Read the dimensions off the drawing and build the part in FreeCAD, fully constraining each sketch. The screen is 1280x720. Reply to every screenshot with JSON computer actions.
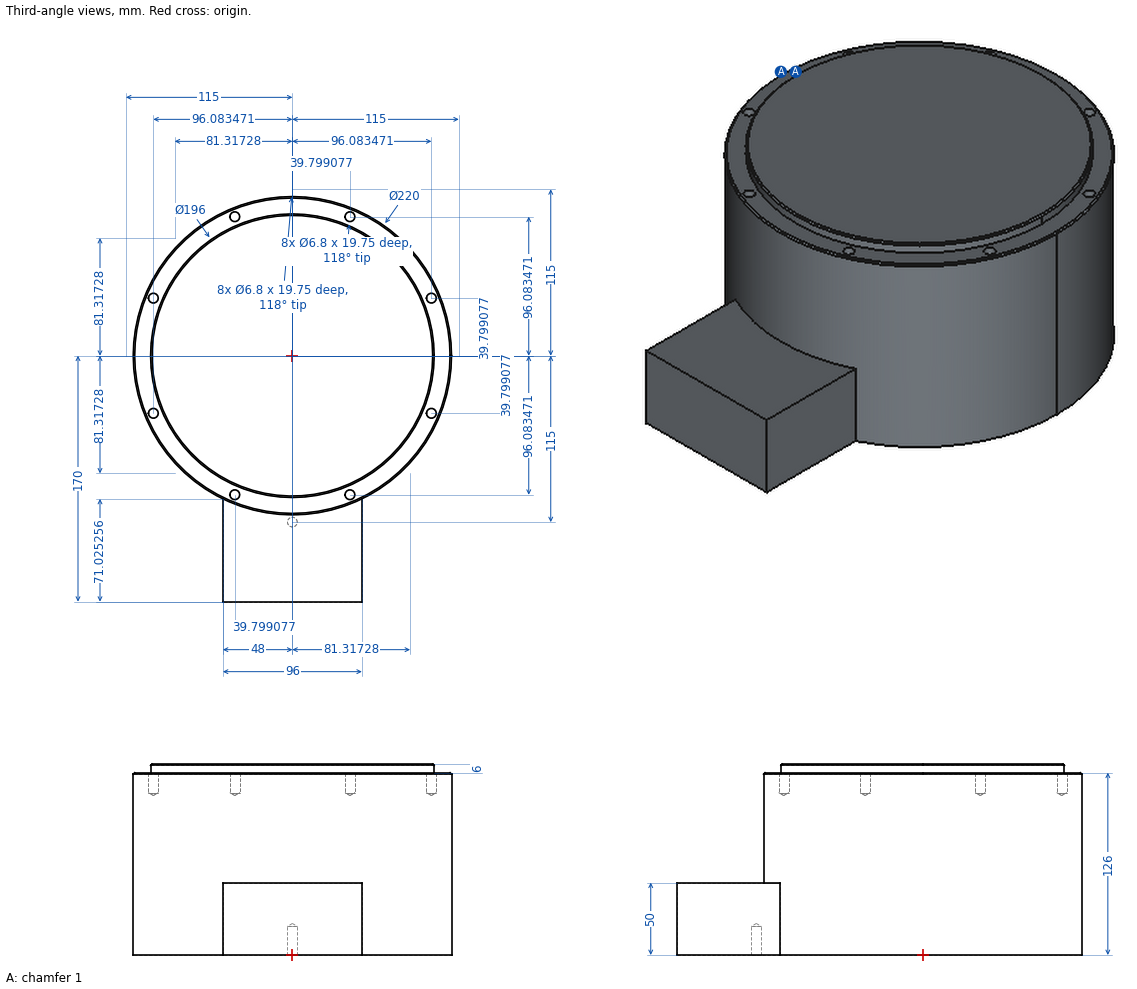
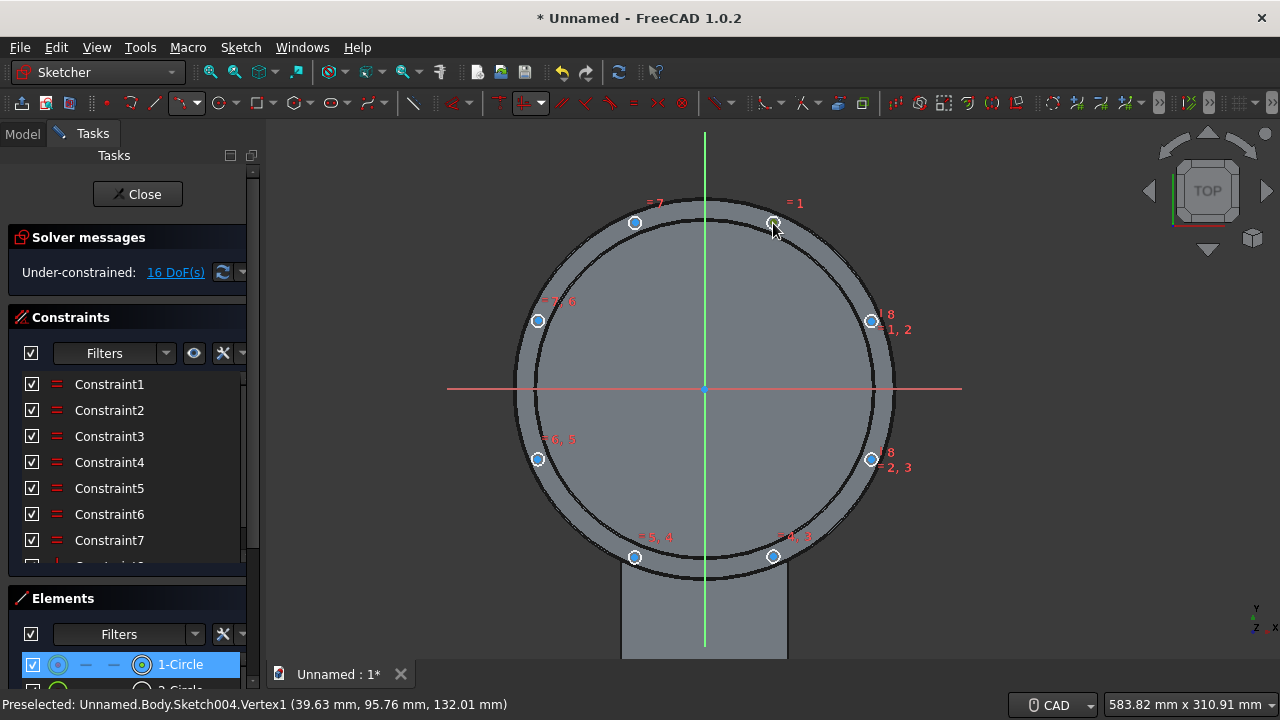
{"action": "left_click", "coordinate": [773, 557]}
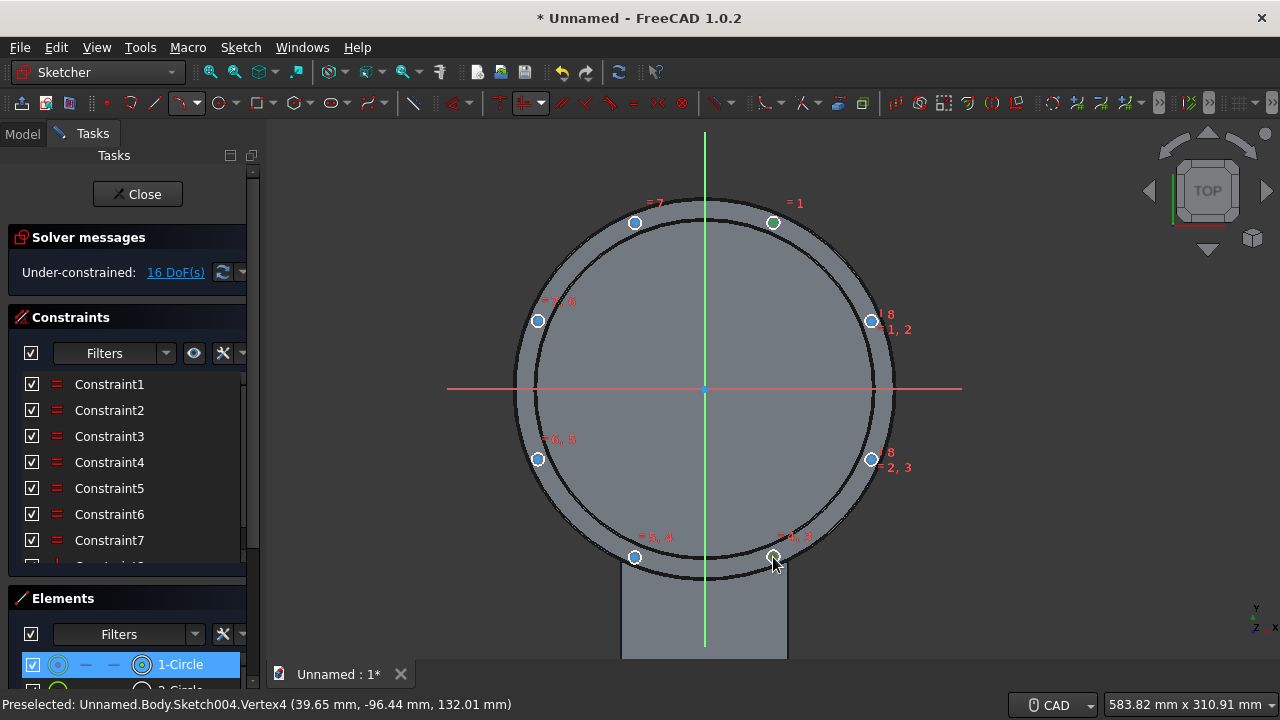
{"action": "left_click", "coordinate": [544, 104]}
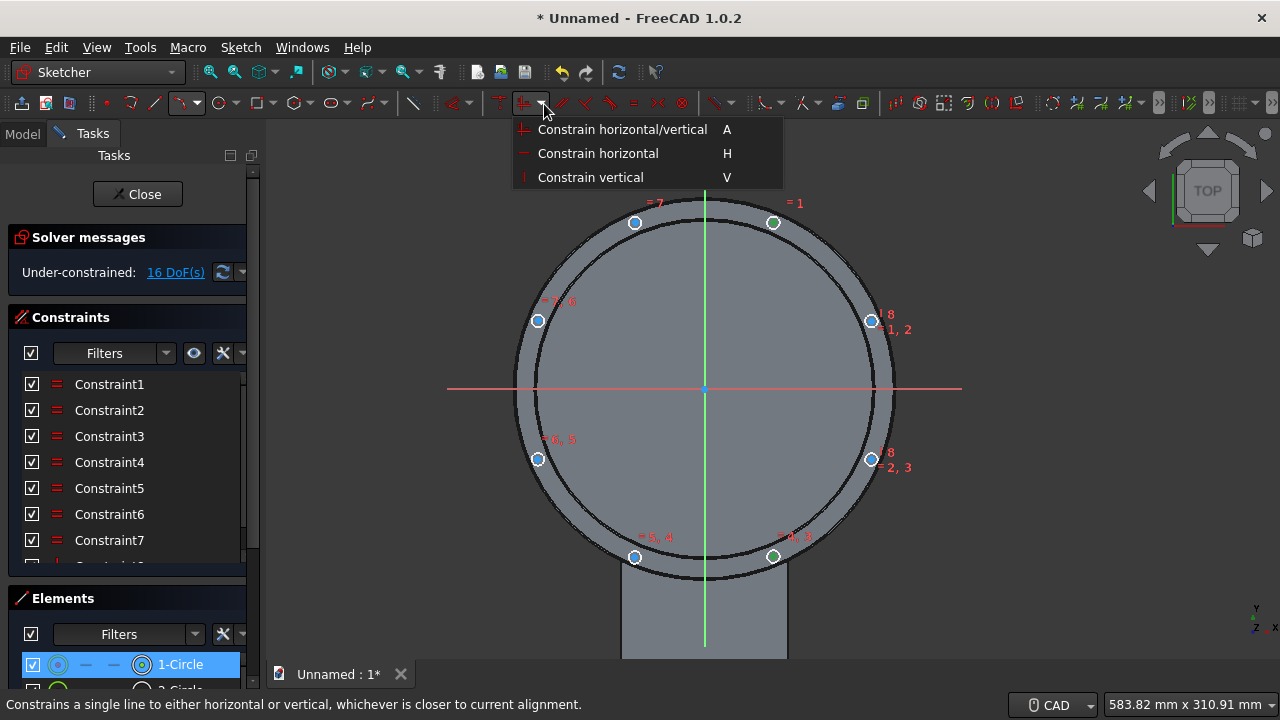
{"action": "left_click", "coordinate": [648, 177]}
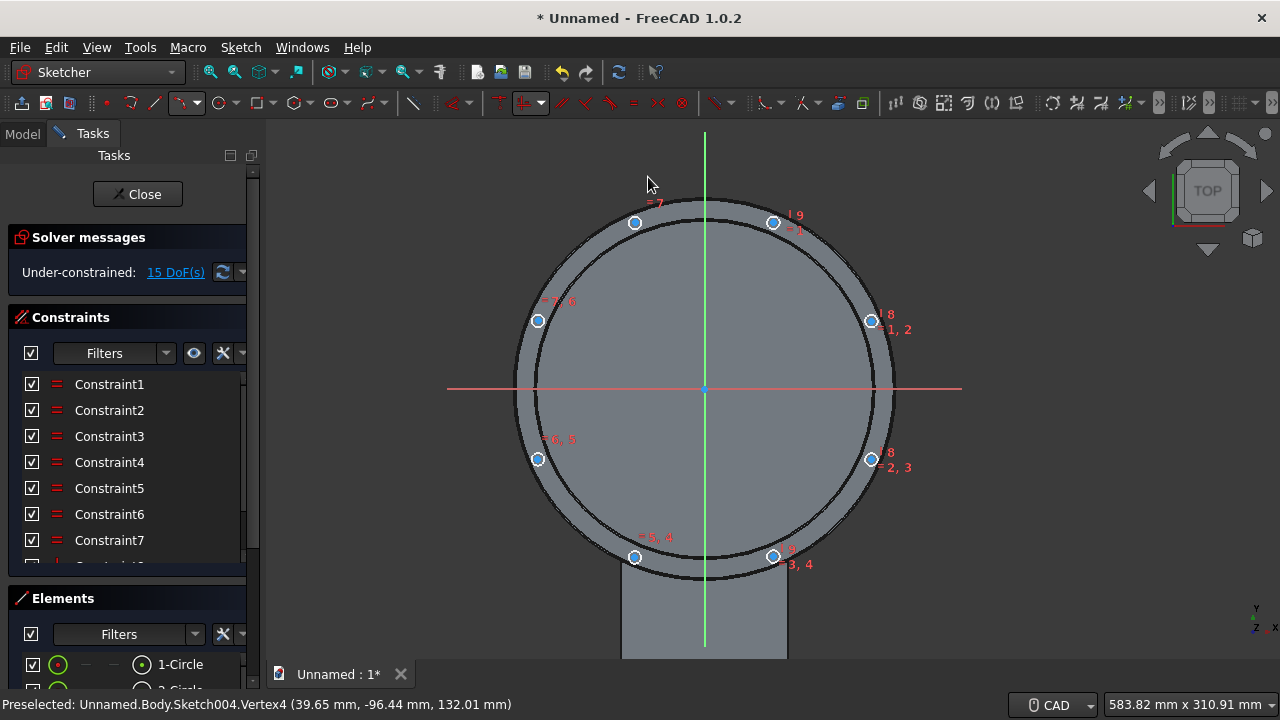
{"action": "left_click", "coordinate": [773, 557]}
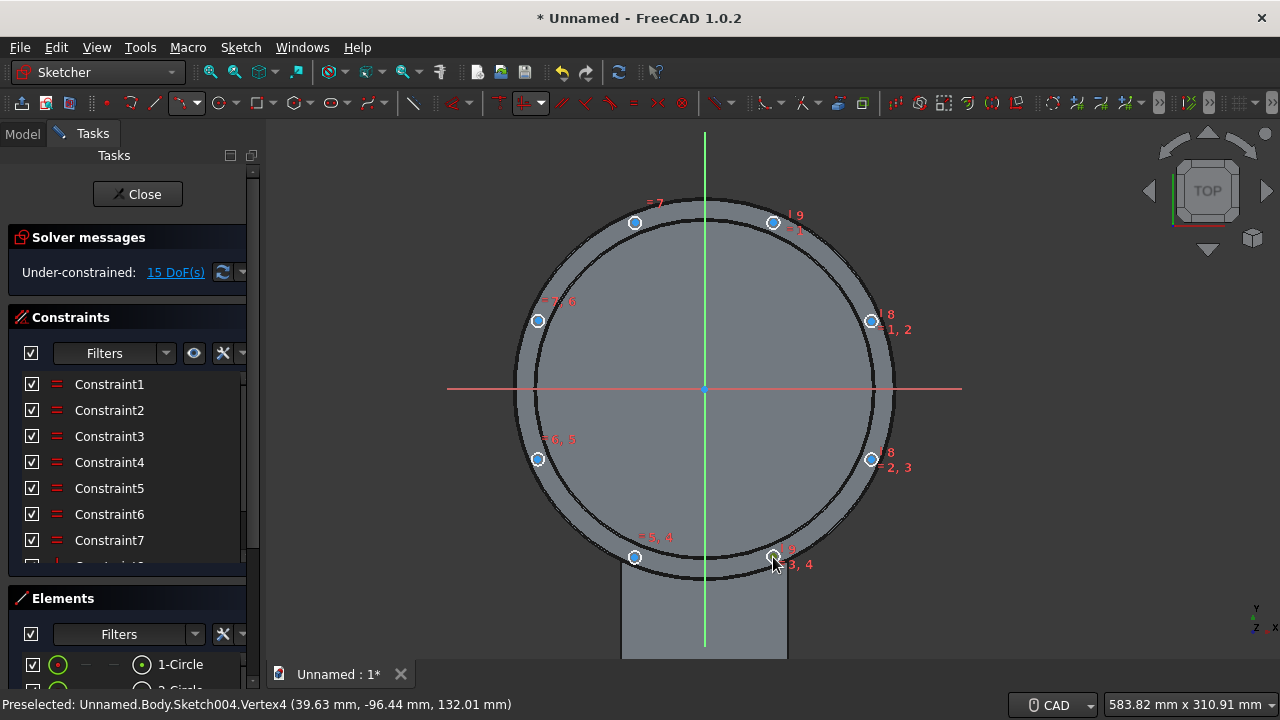
{"action": "left_click", "coordinate": [635, 557]}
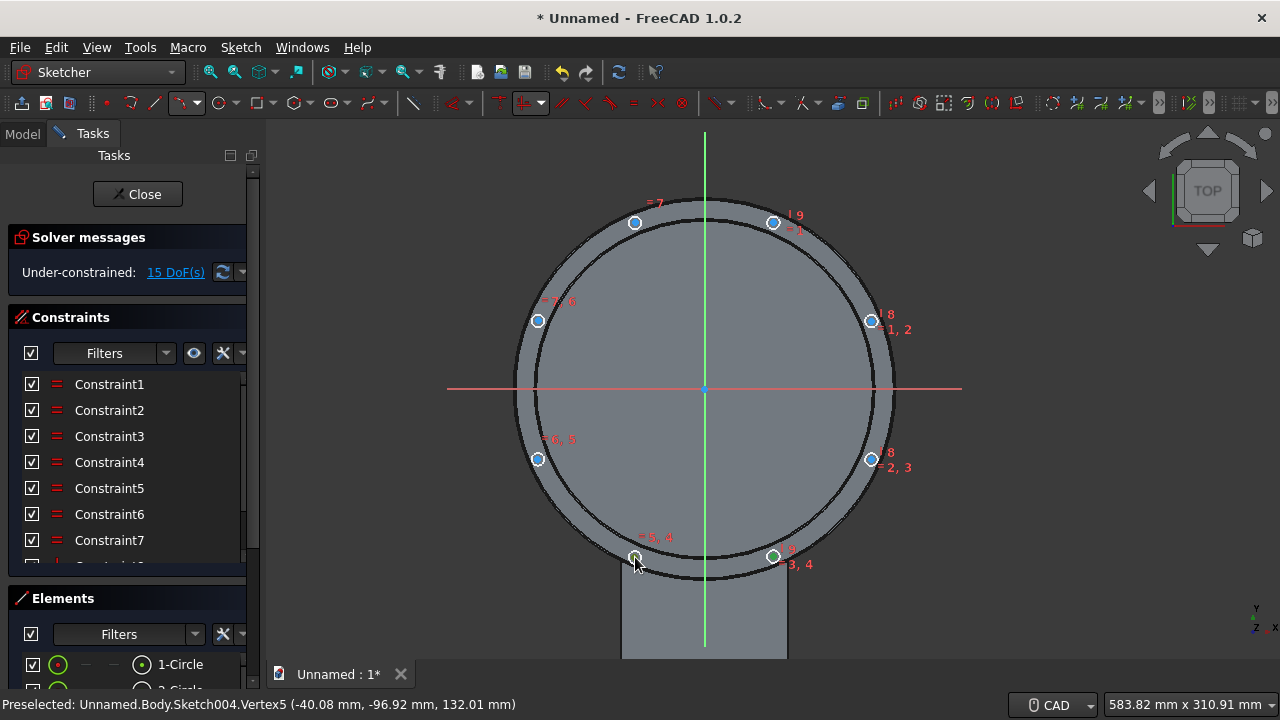
{"action": "left_click", "coordinate": [544, 104]}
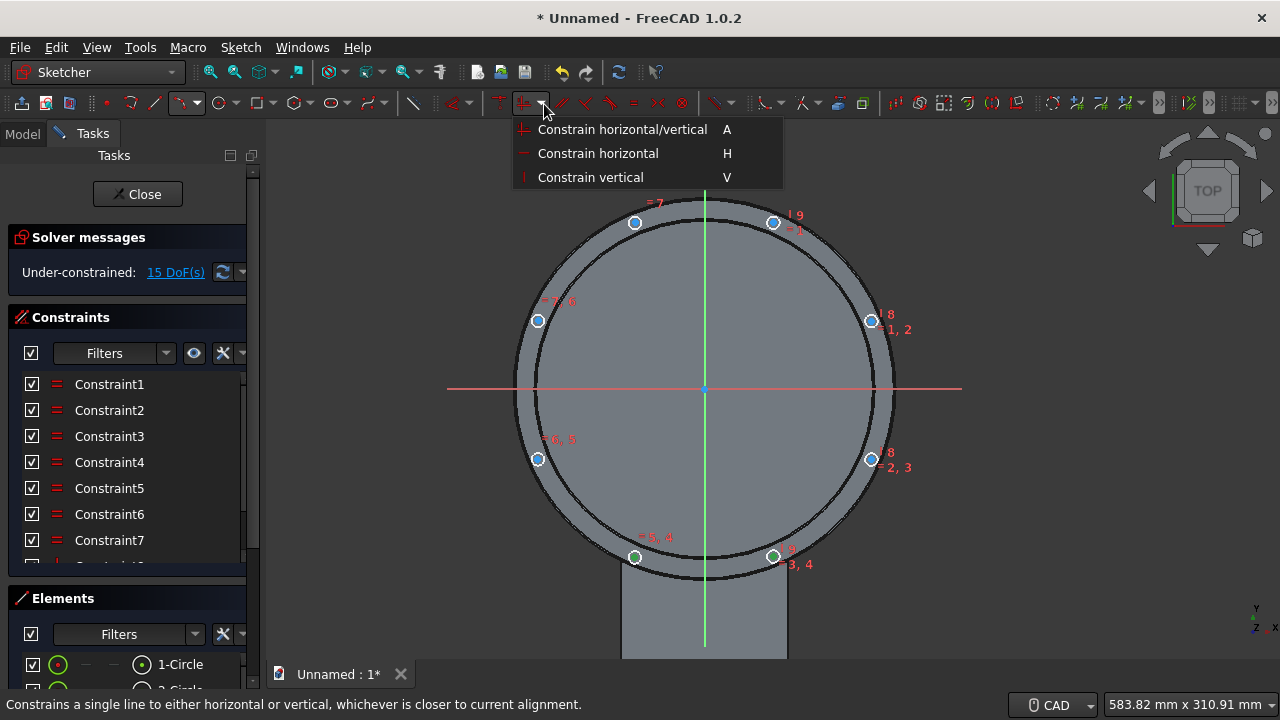
{"action": "left_click", "coordinate": [648, 153]}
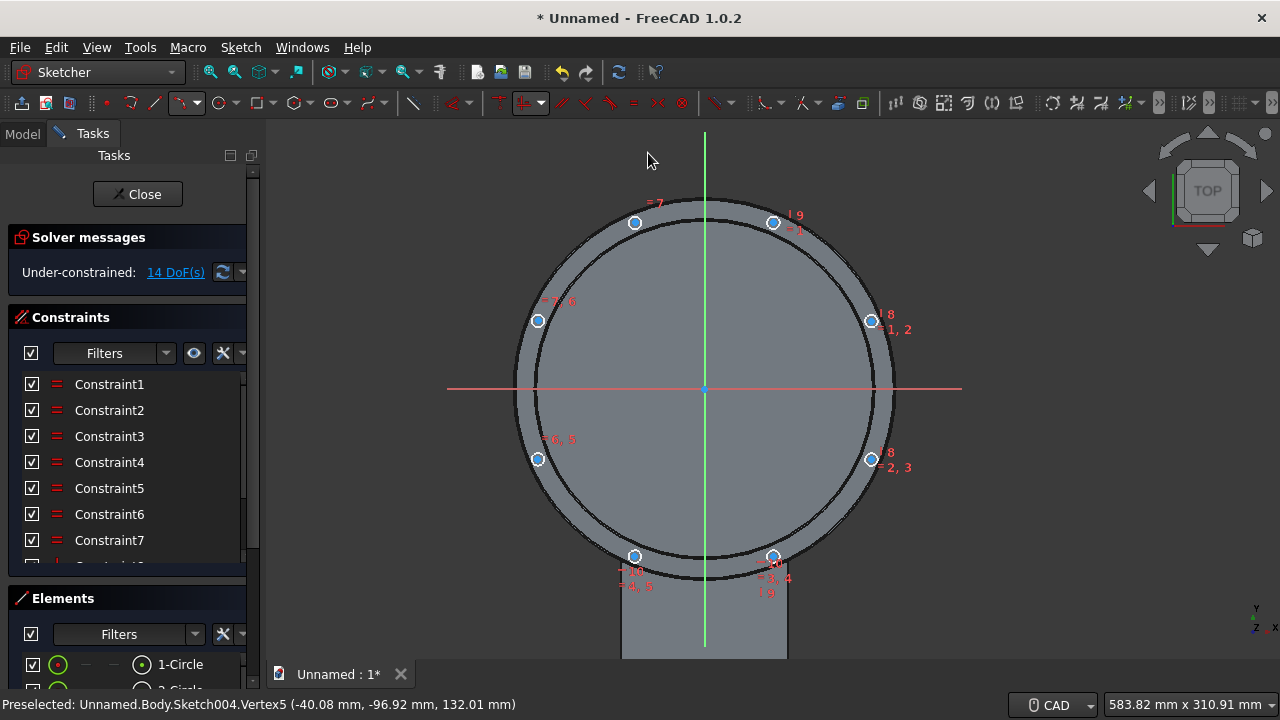
{"action": "left_click", "coordinate": [871, 460]}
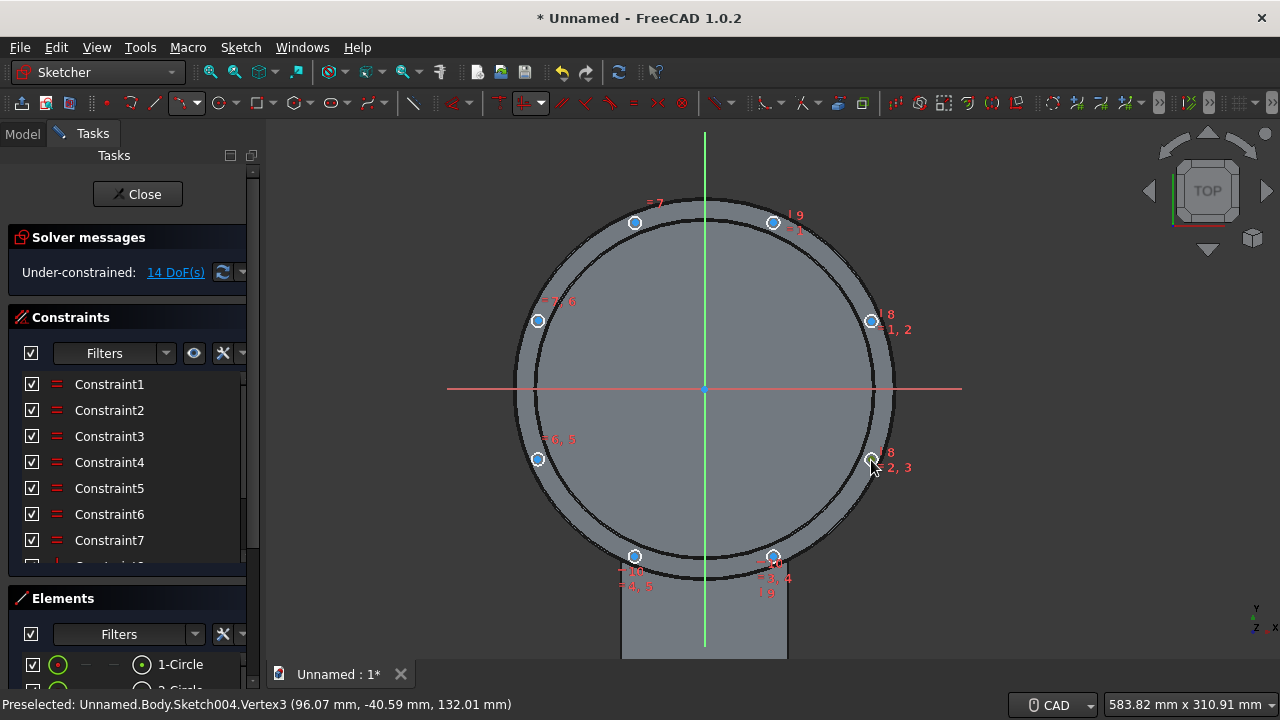
{"action": "left_click", "coordinate": [538, 459]}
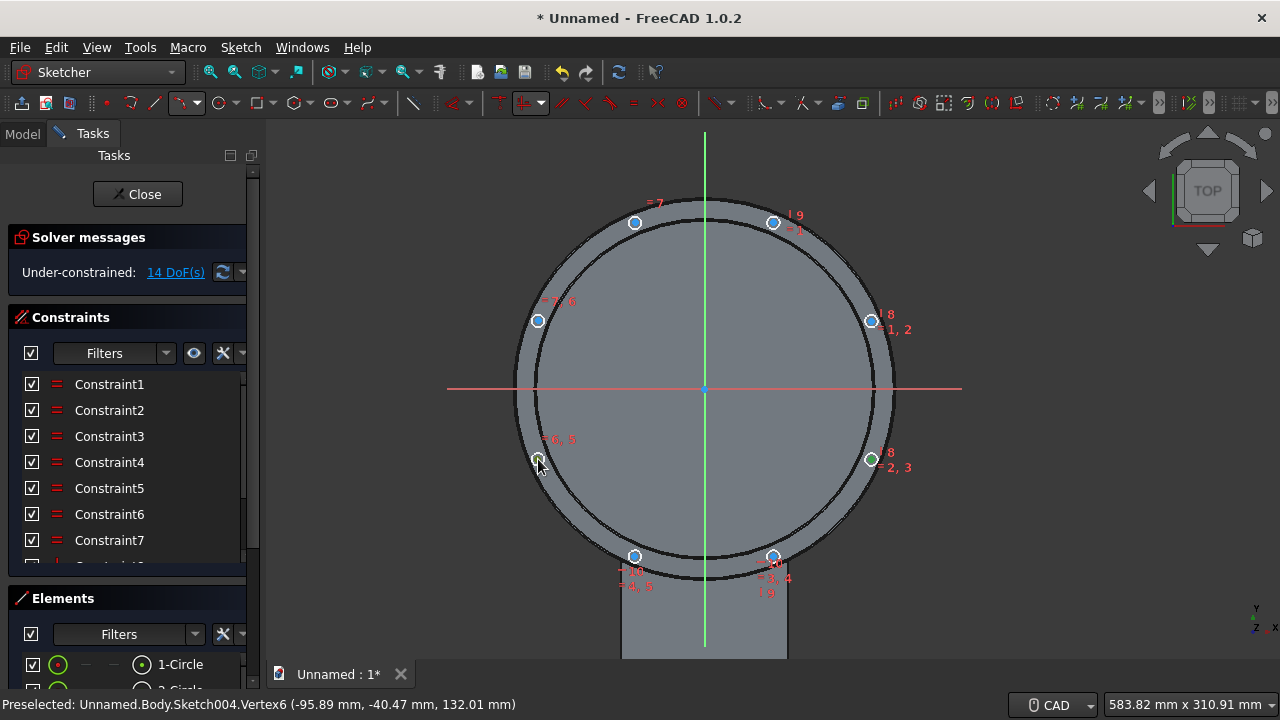
{"action": "key", "text": "h"}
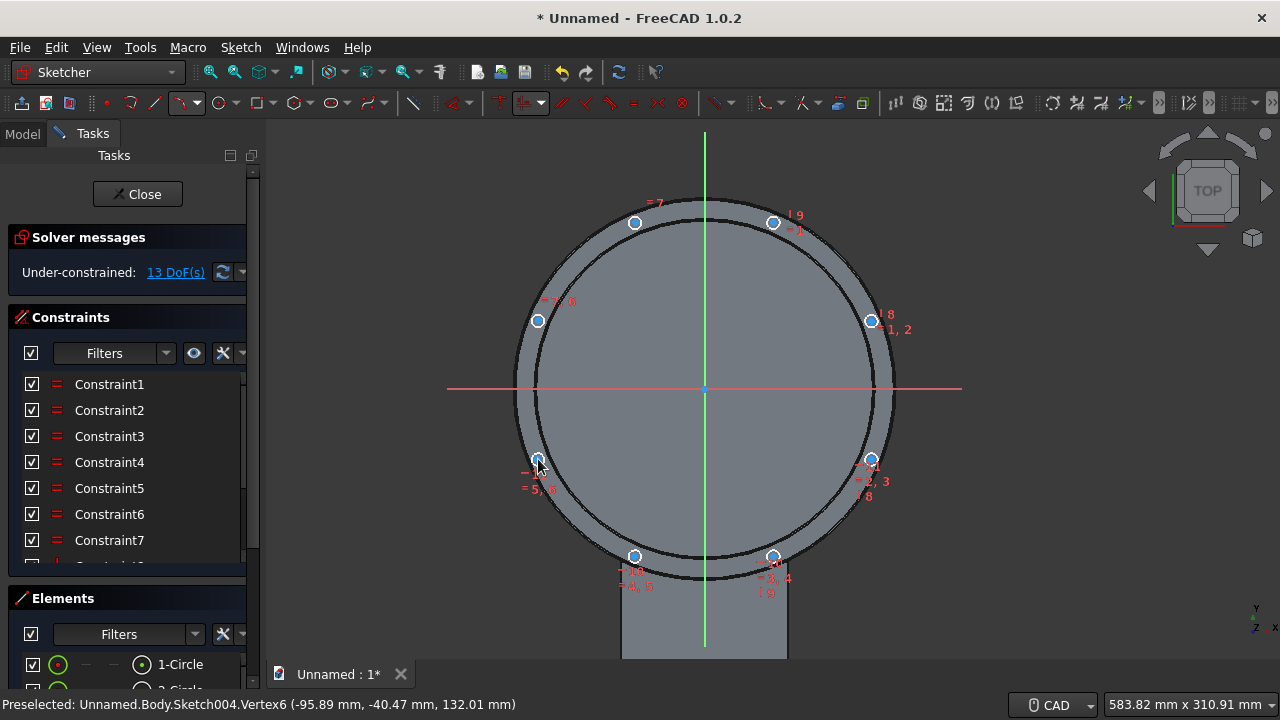
{"action": "left_click", "coordinate": [538, 460]}